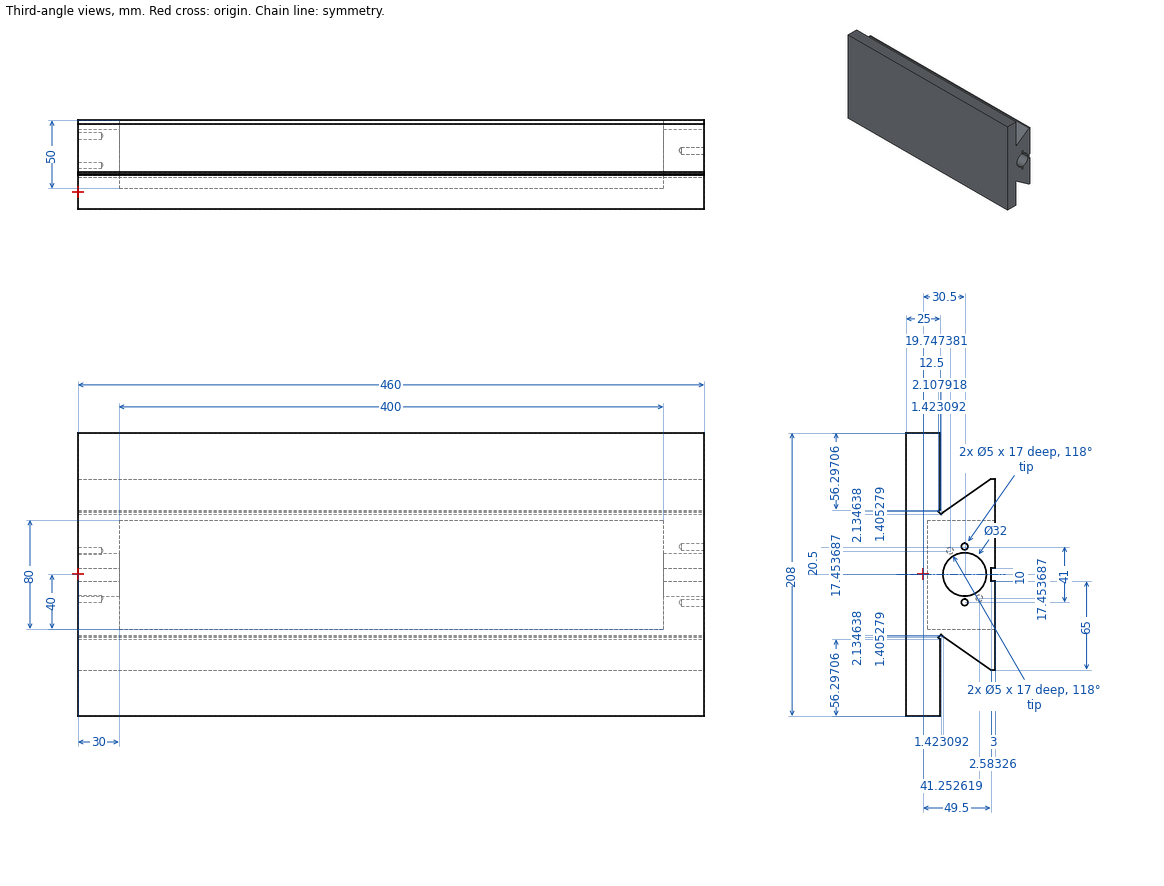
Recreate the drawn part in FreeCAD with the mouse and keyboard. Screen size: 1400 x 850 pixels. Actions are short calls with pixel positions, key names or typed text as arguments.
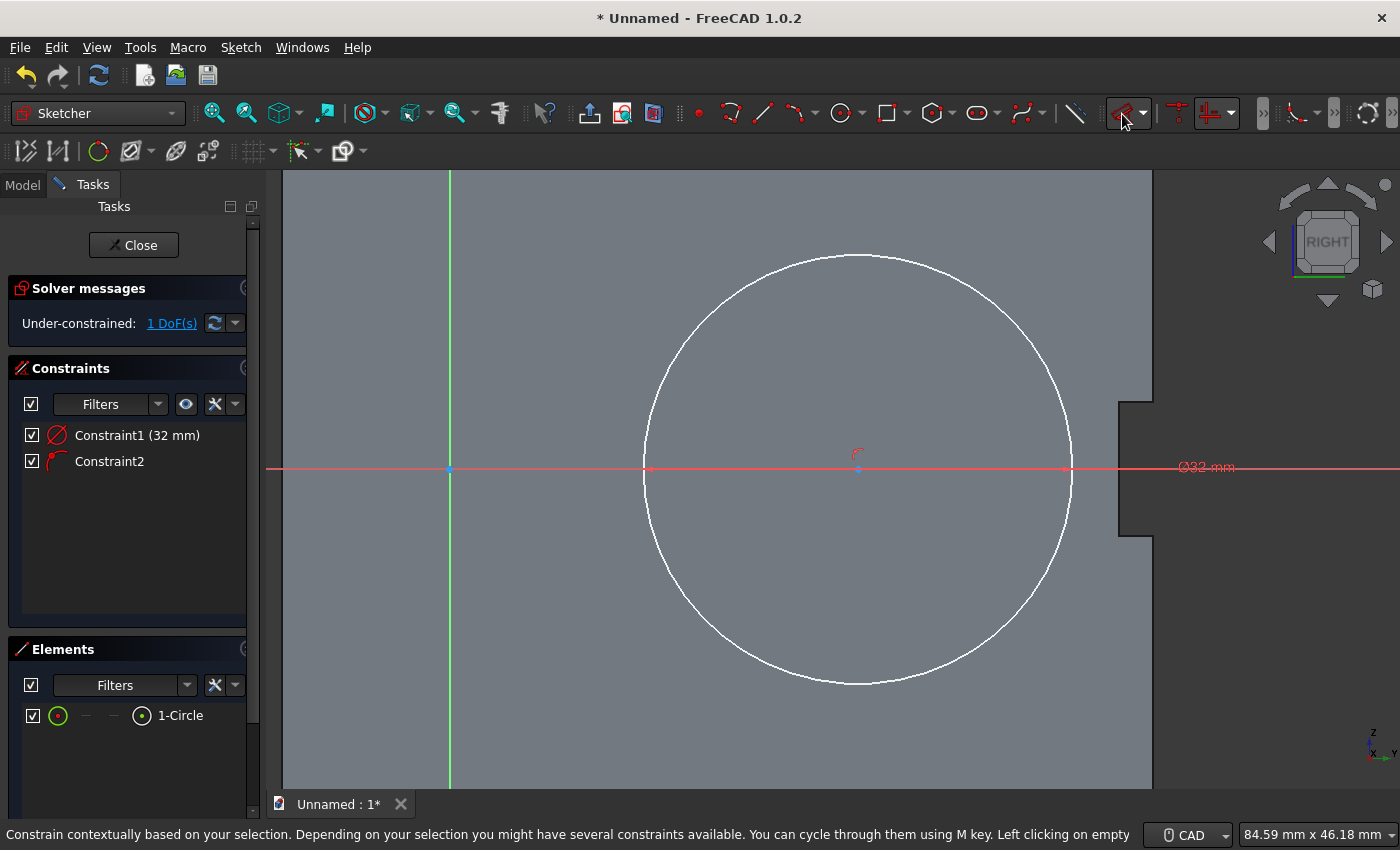
click(858, 469)
click(560, 503)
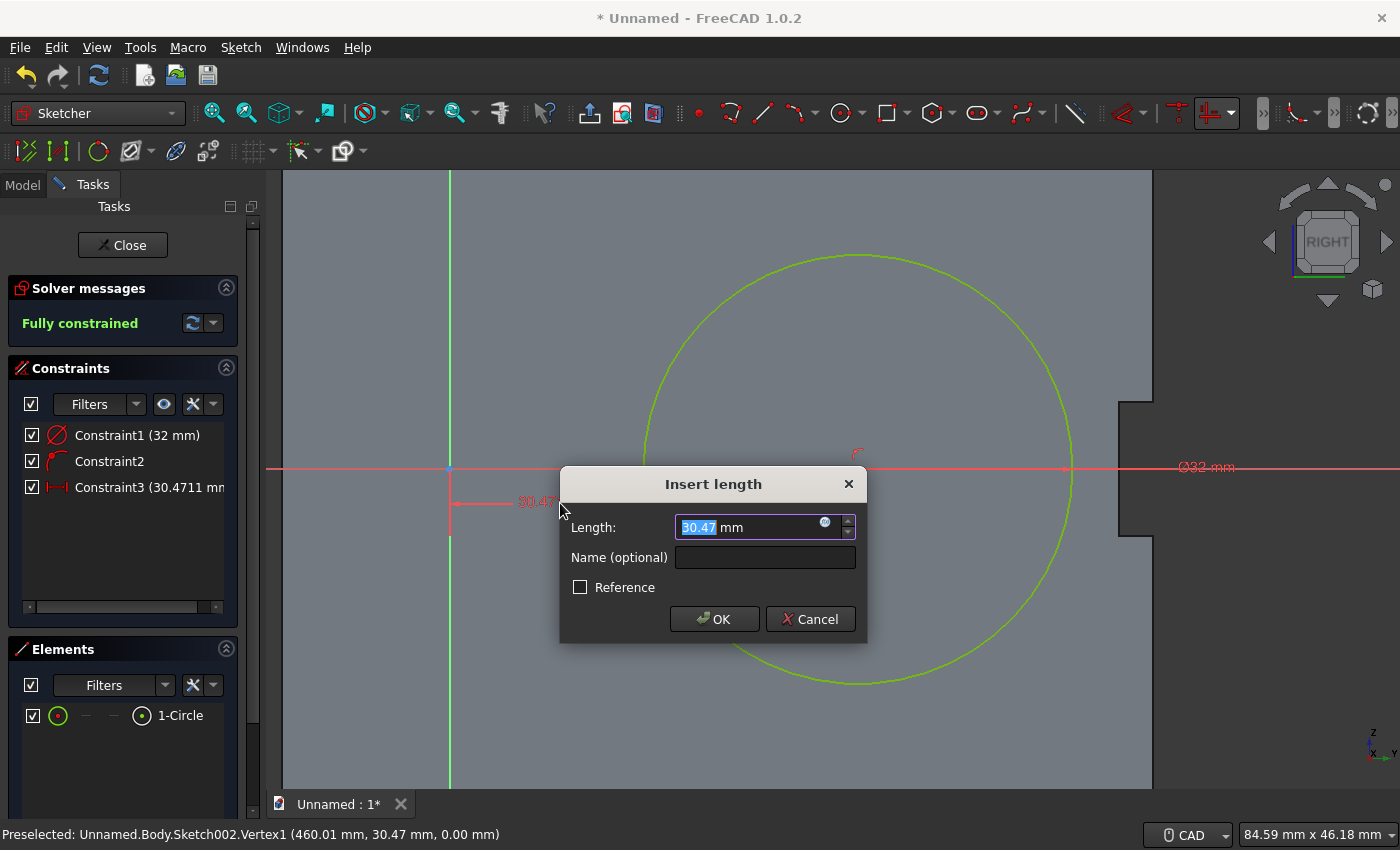
text(30.5)
key(Return)
key(Escape)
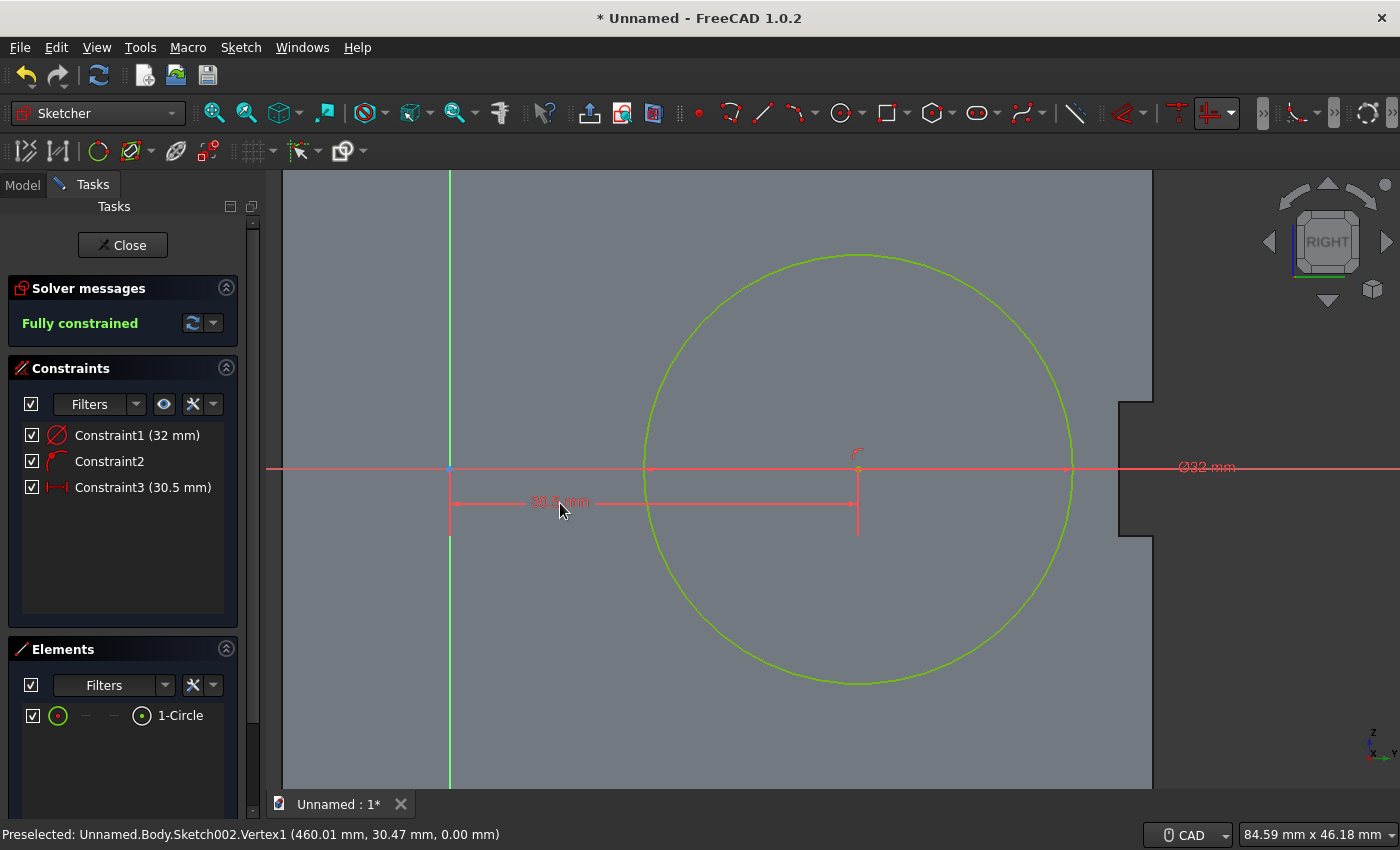
click(123, 245)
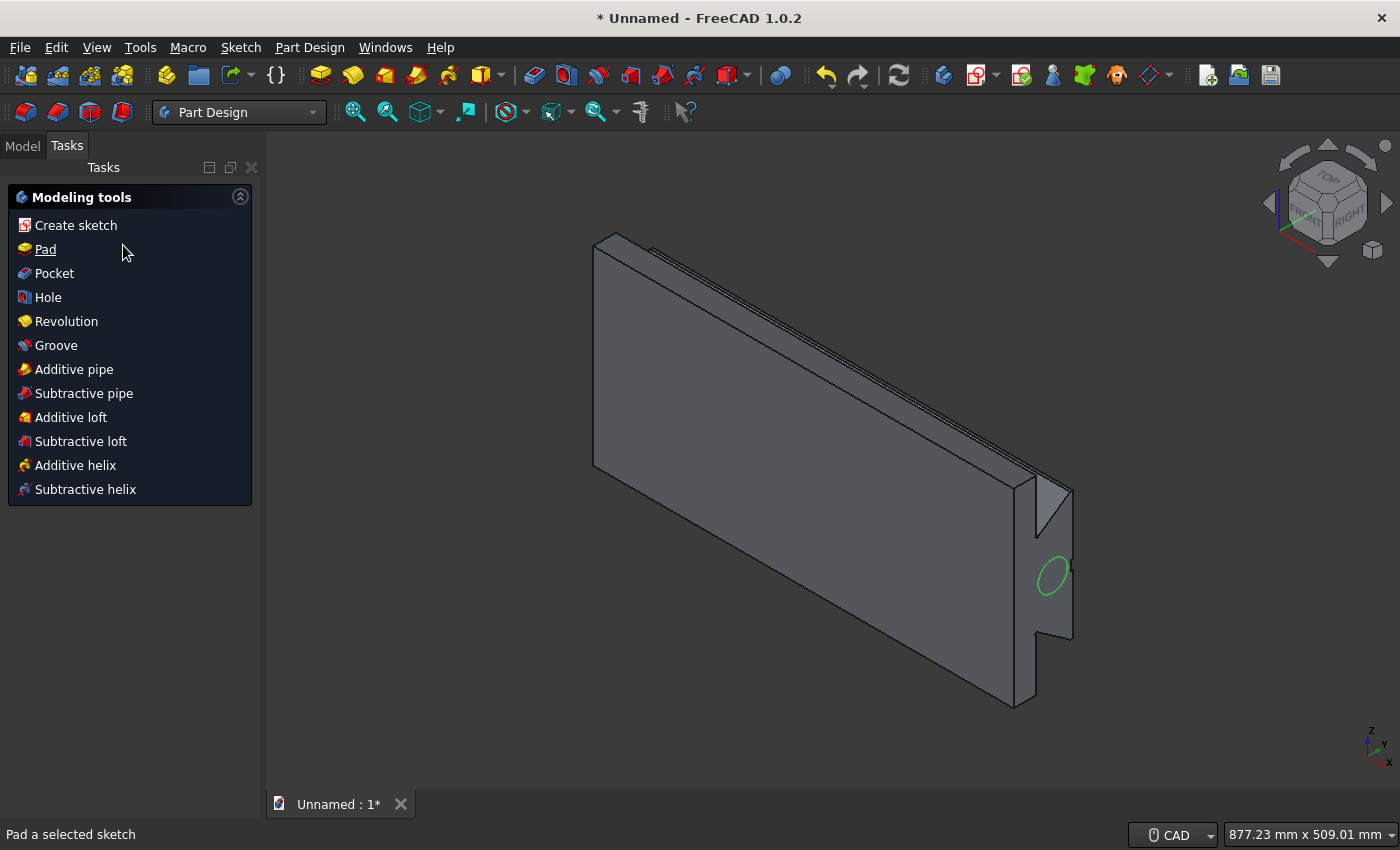
click(536, 76)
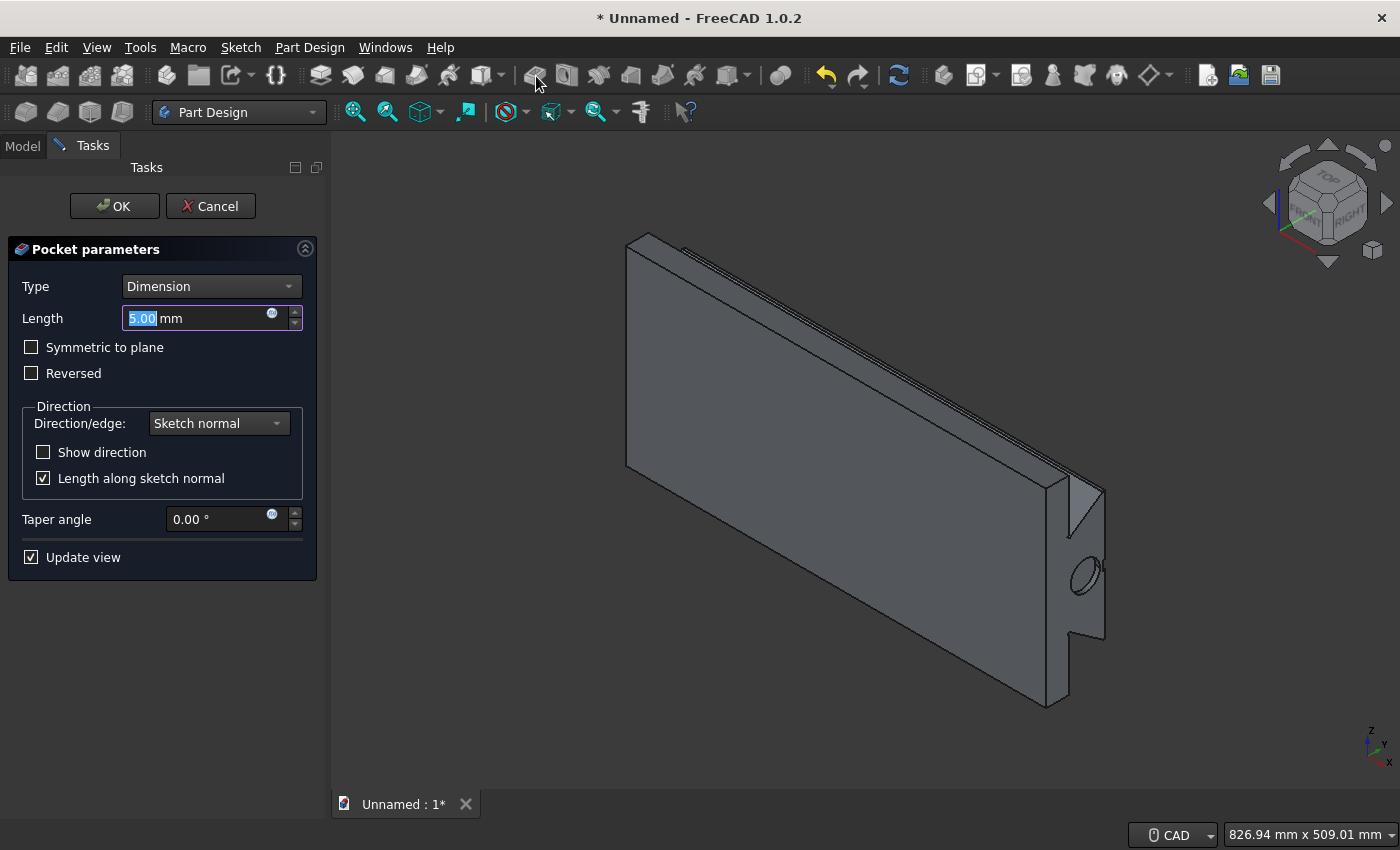
click(212, 286)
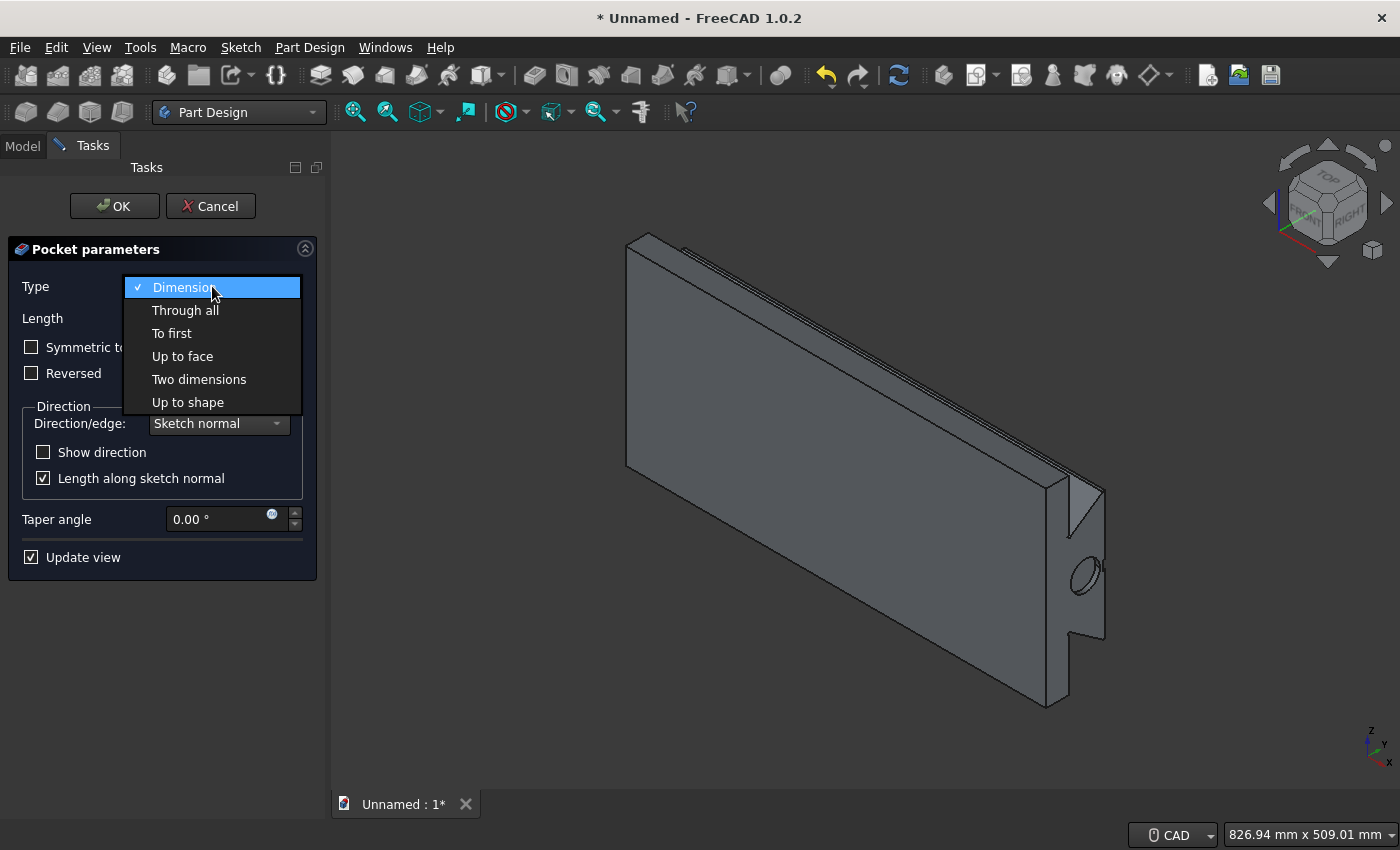
click(212, 310)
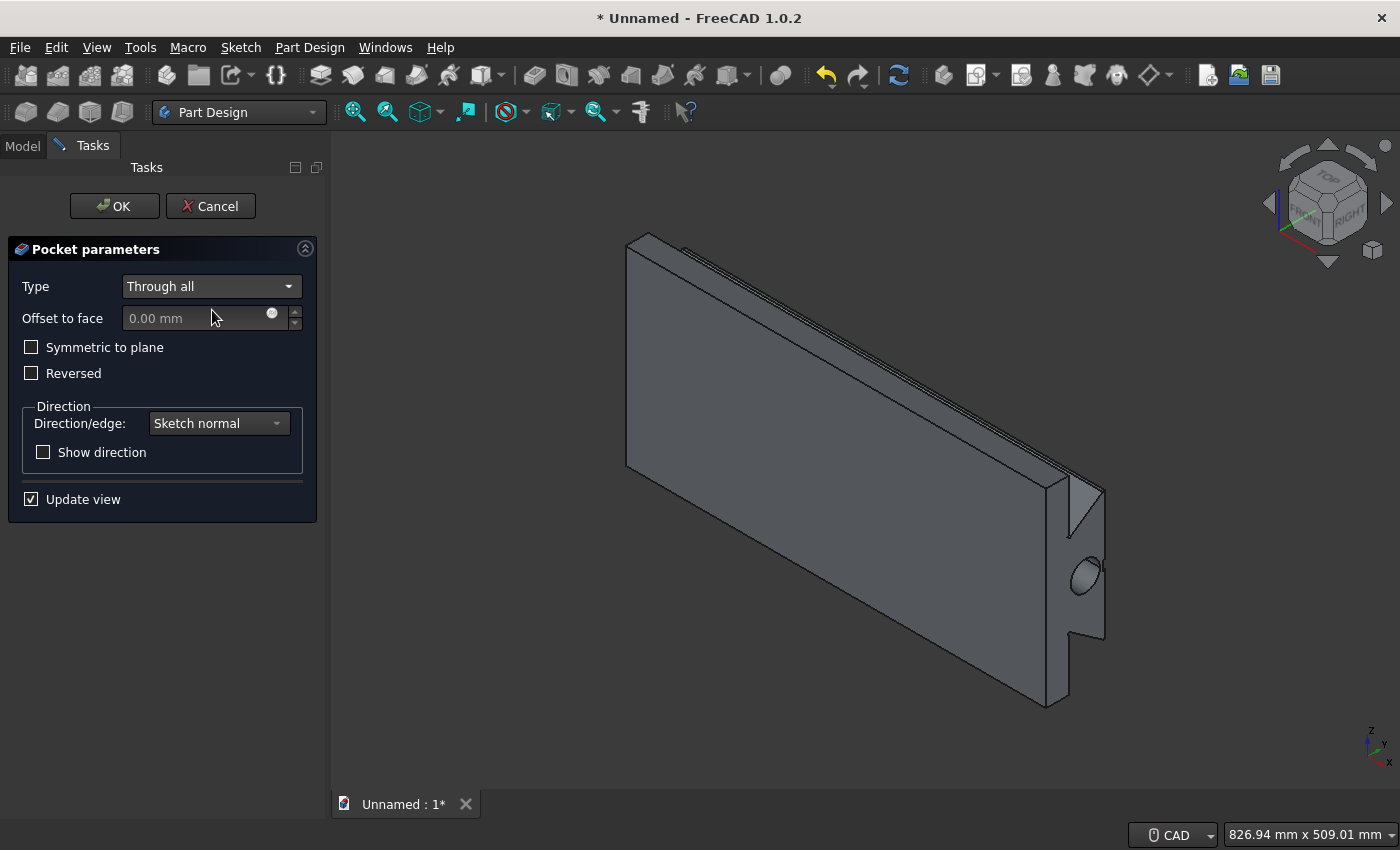
click(115, 206)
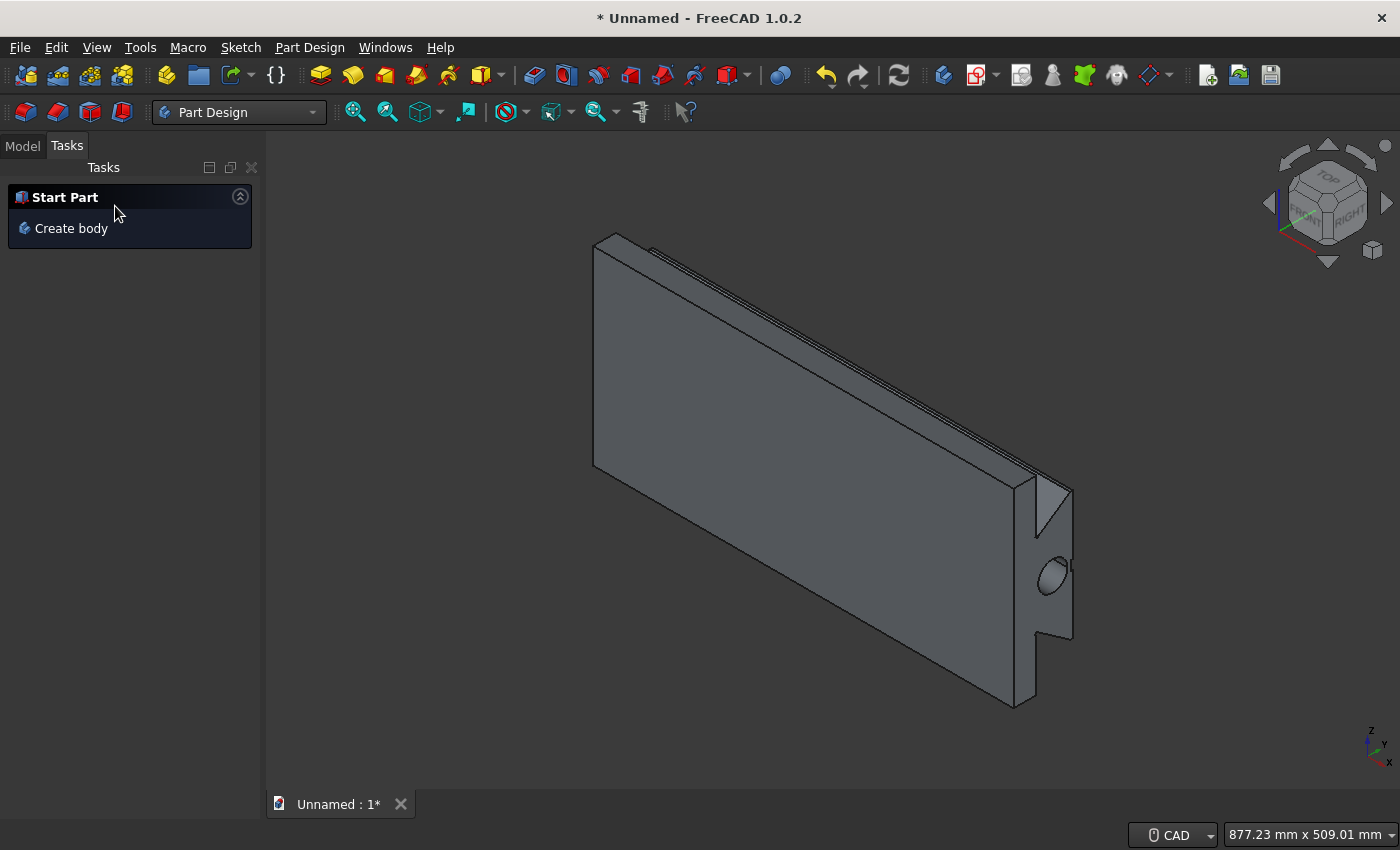
click(1043, 612)